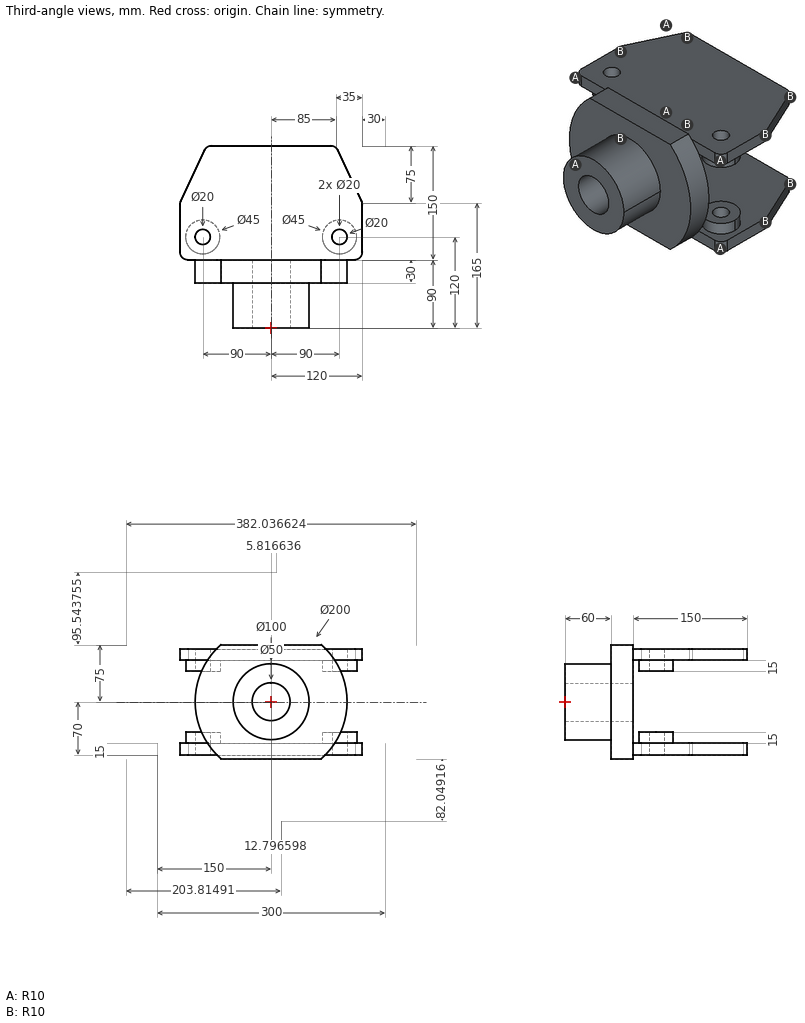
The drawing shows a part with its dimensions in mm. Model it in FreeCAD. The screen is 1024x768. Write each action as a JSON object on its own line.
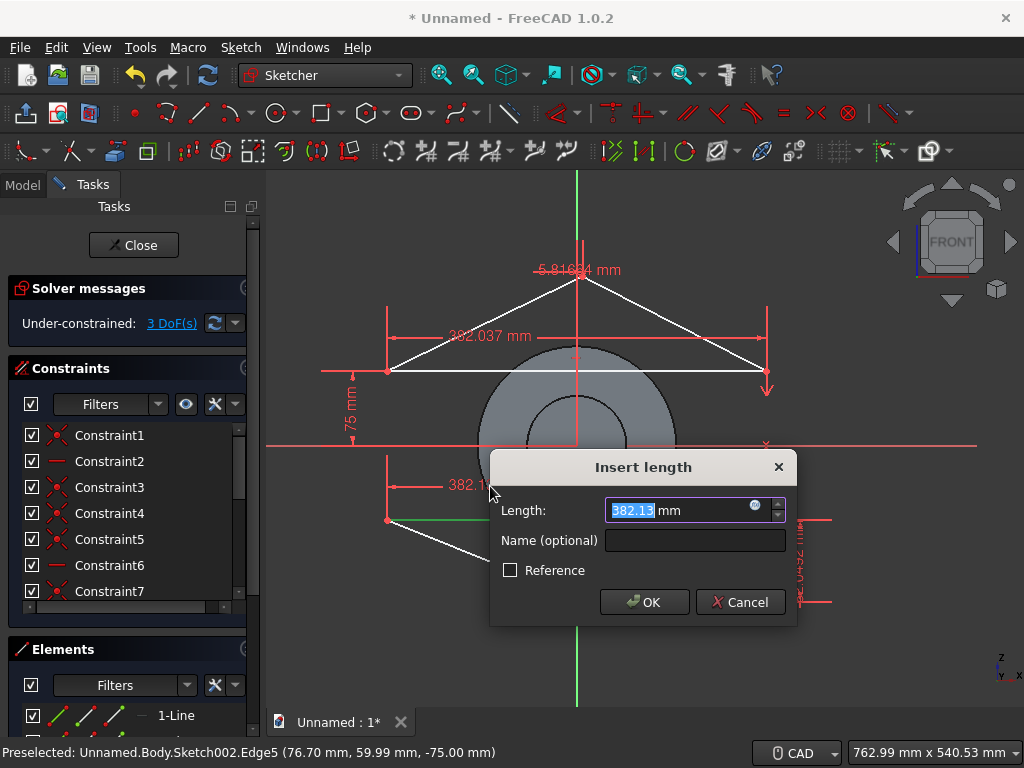
{"action": "type", "text": "382.036624"}
{"action": "key", "text": "Return"}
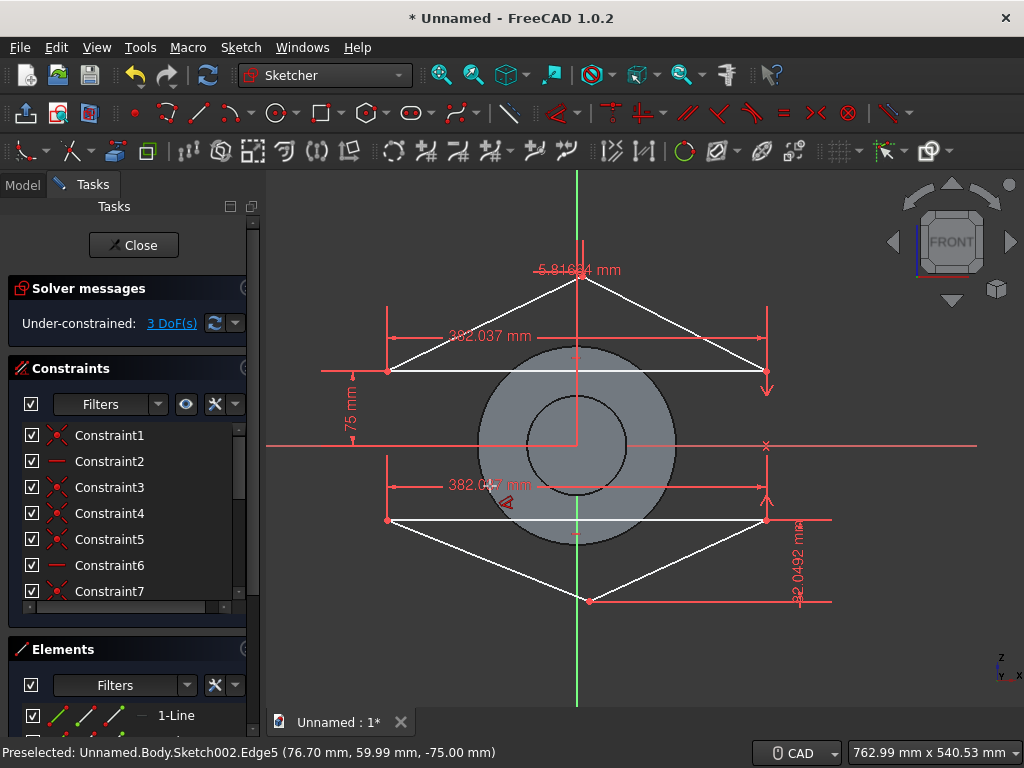
{"action": "scroll", "coordinate": [589, 602], "scroll_direction": "up", "scroll_amount": 6}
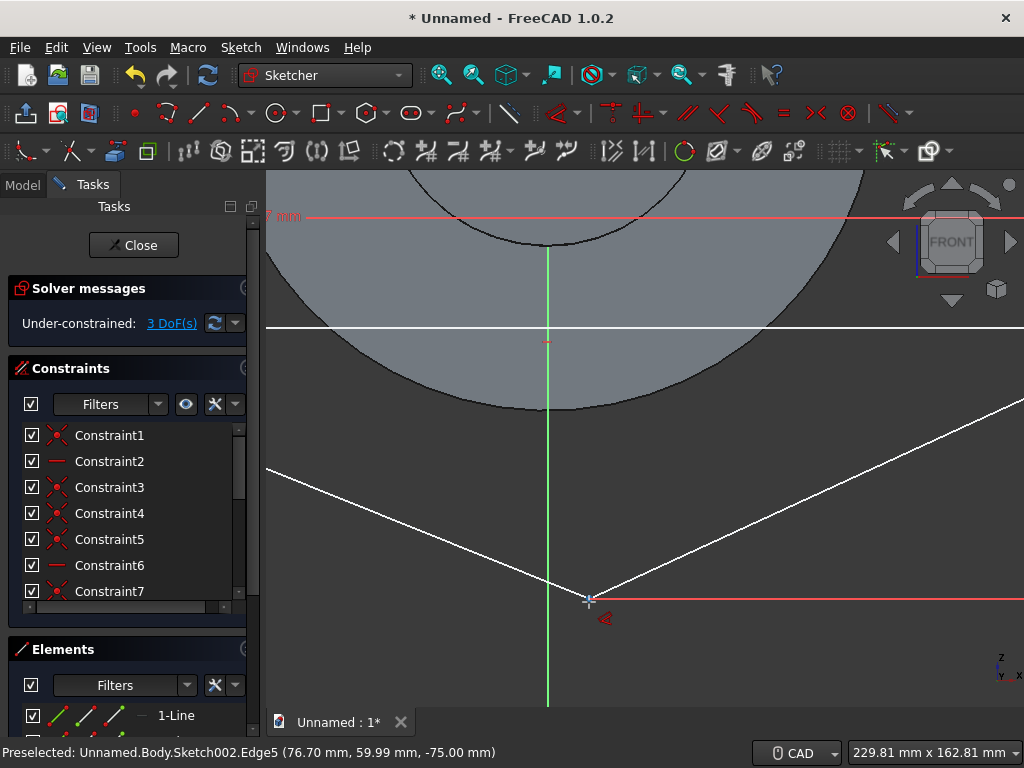
{"action": "left_click", "coordinate": [590, 599]}
{"action": "left_click", "coordinate": [569, 633]}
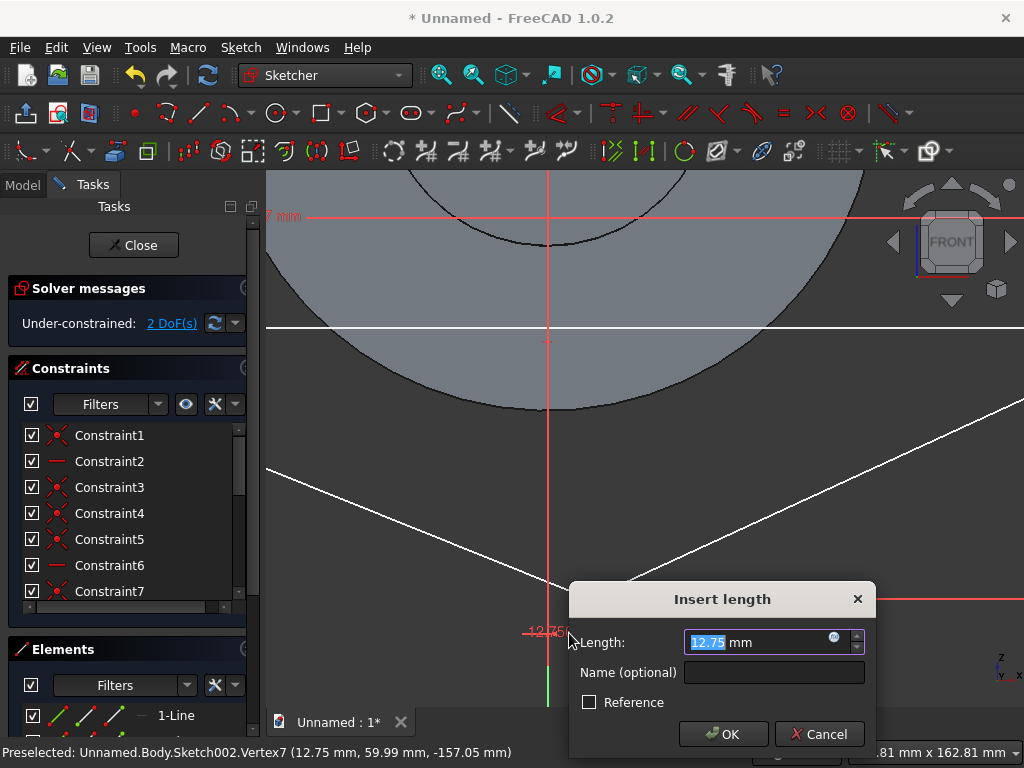
{"action": "type", "text": "12.796598"}
{"action": "key", "text": "Return"}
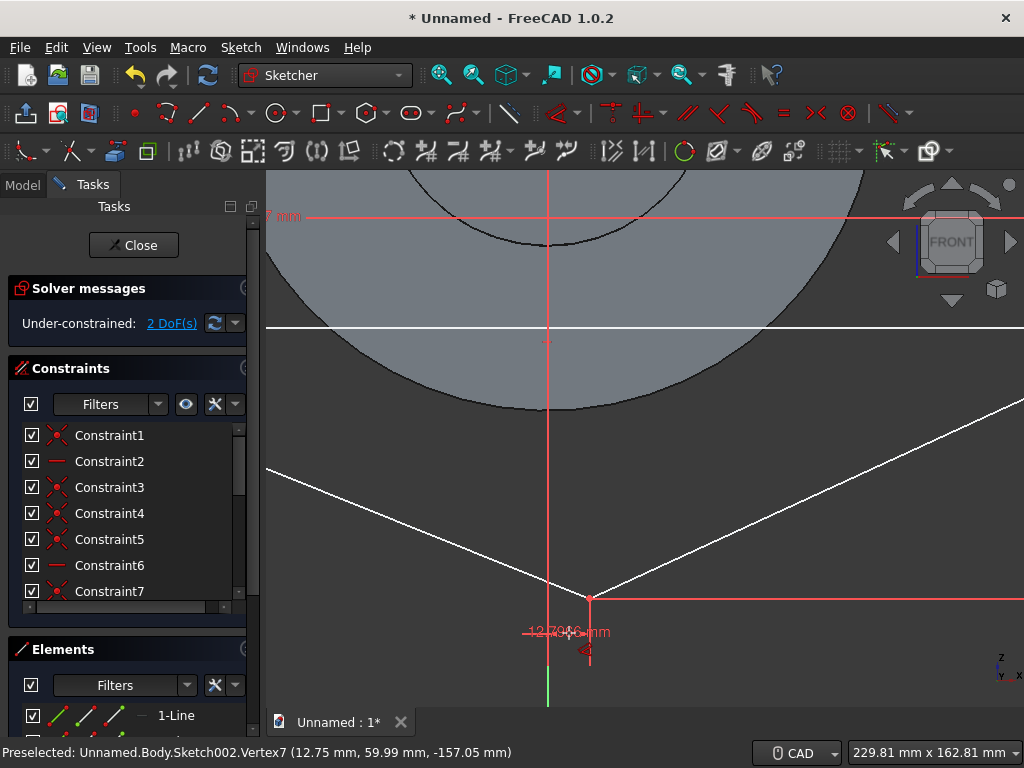
{"action": "scroll", "coordinate": [589, 602], "scroll_direction": "down", "scroll_amount": 6}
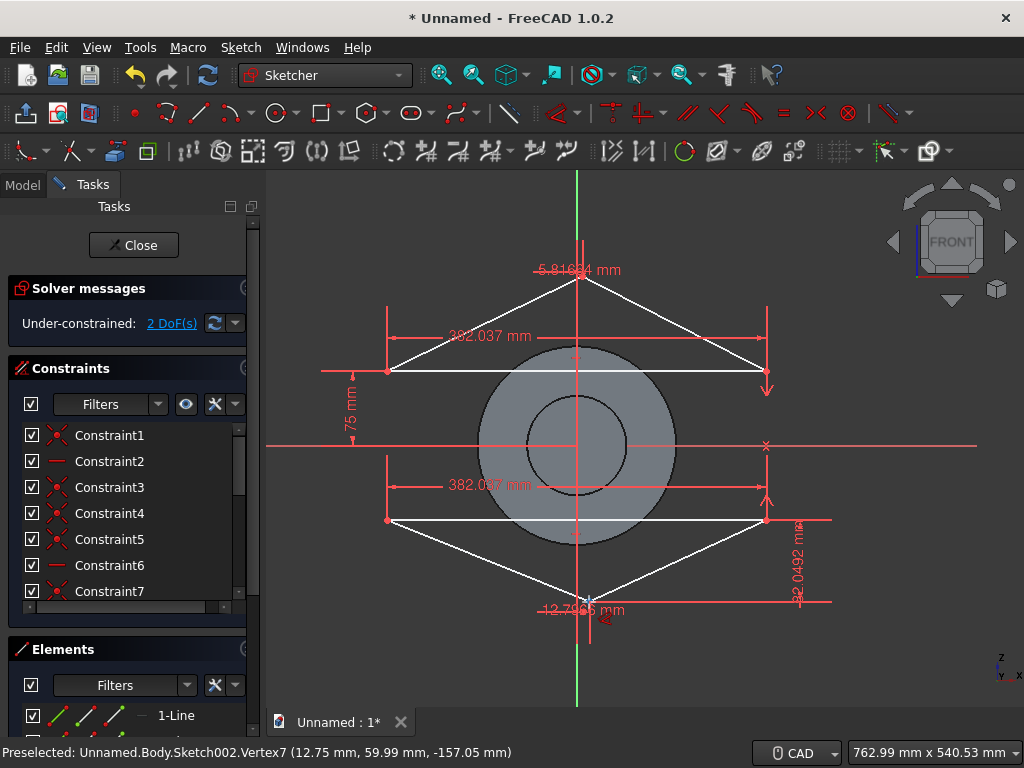
{"action": "left_click", "coordinate": [524, 305]}
{"action": "left_click", "coordinate": [353, 324]}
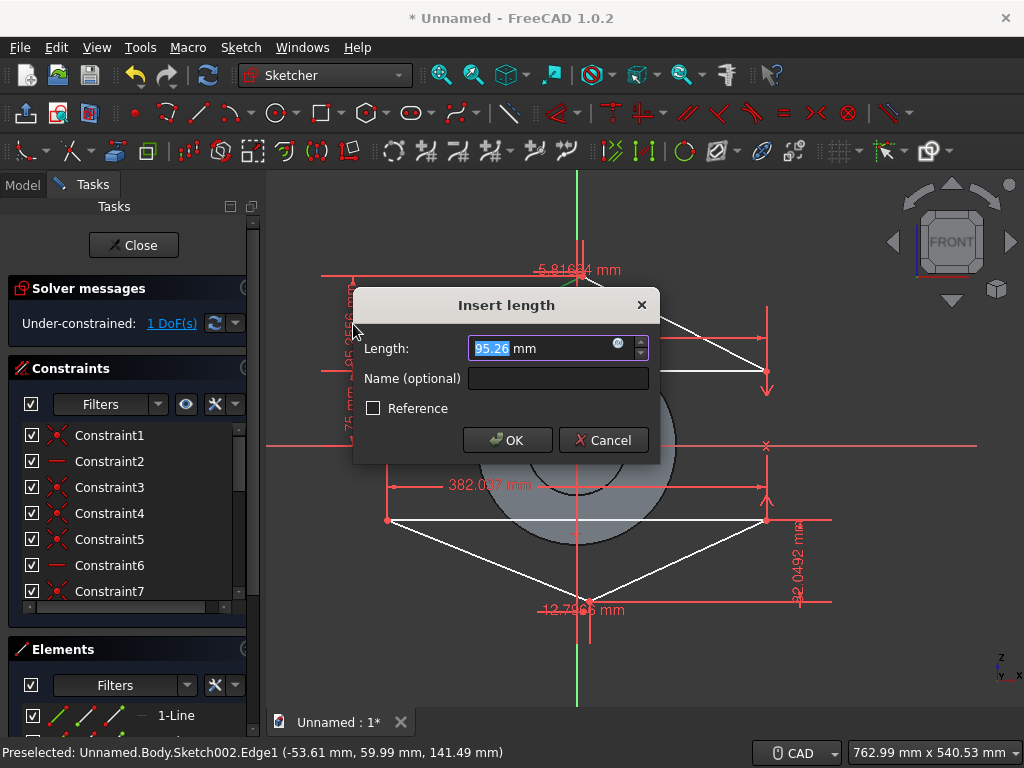
{"action": "type", "text": "95.543755"}
{"action": "key", "text": "Return"}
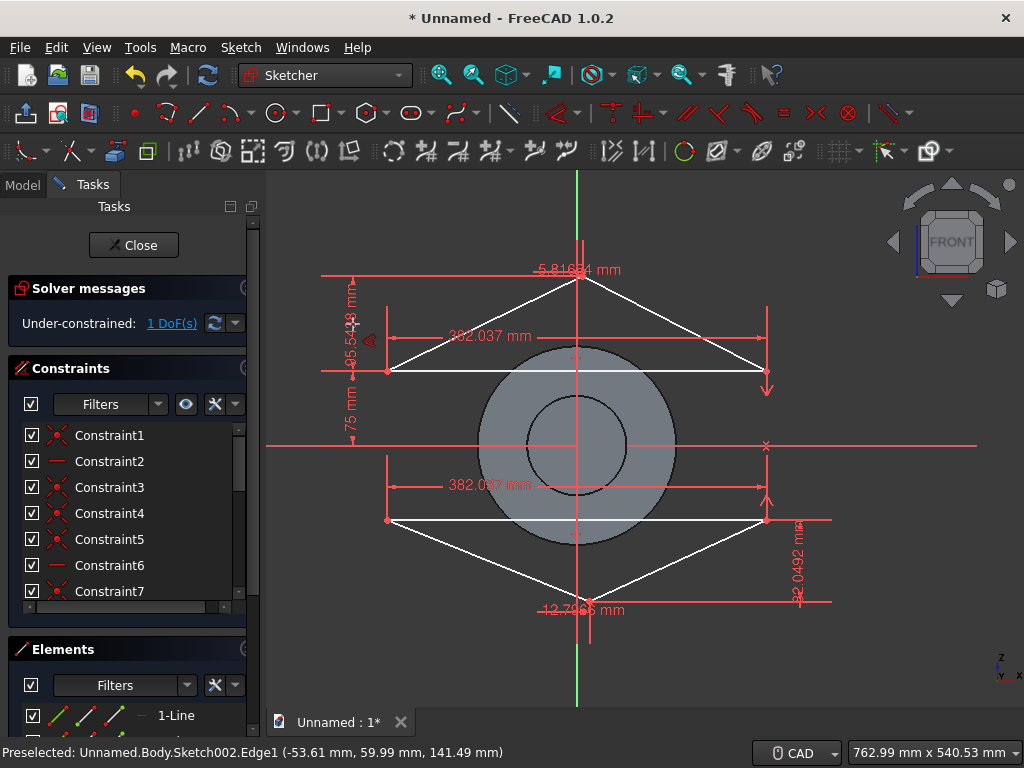
{"action": "left_click", "coordinate": [448, 545]}
{"action": "left_click", "coordinate": [488, 636]}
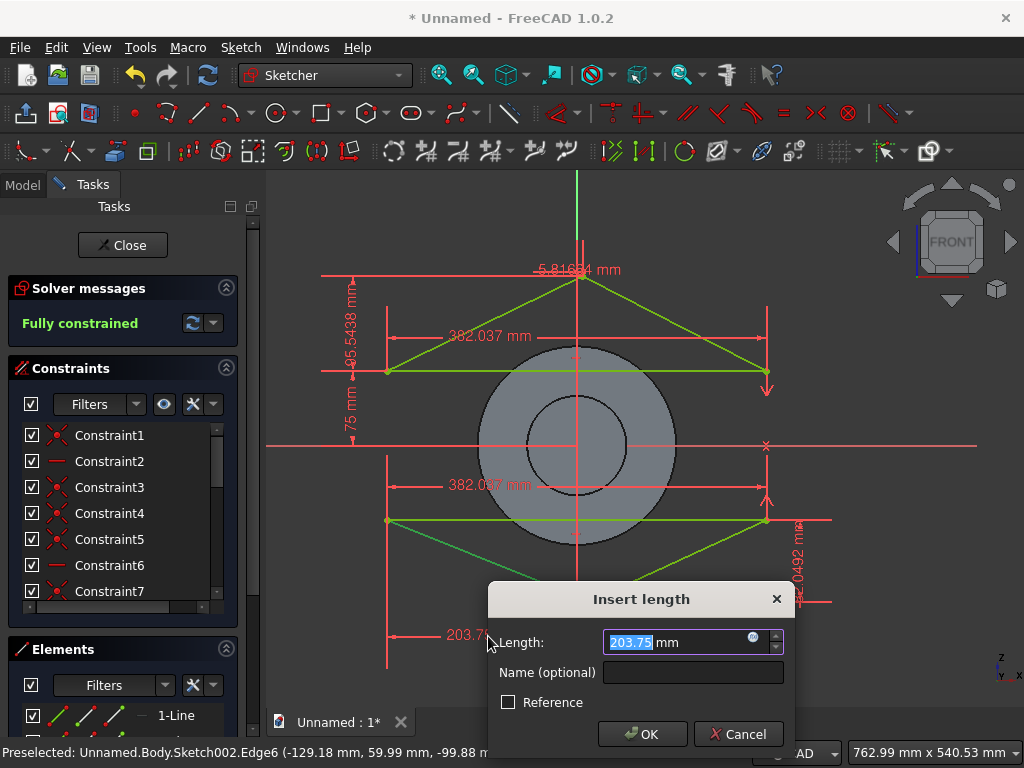
{"action": "type", "text": "203.81491"}
{"action": "key", "text": "Return"}
{"action": "key", "text": "Escape"}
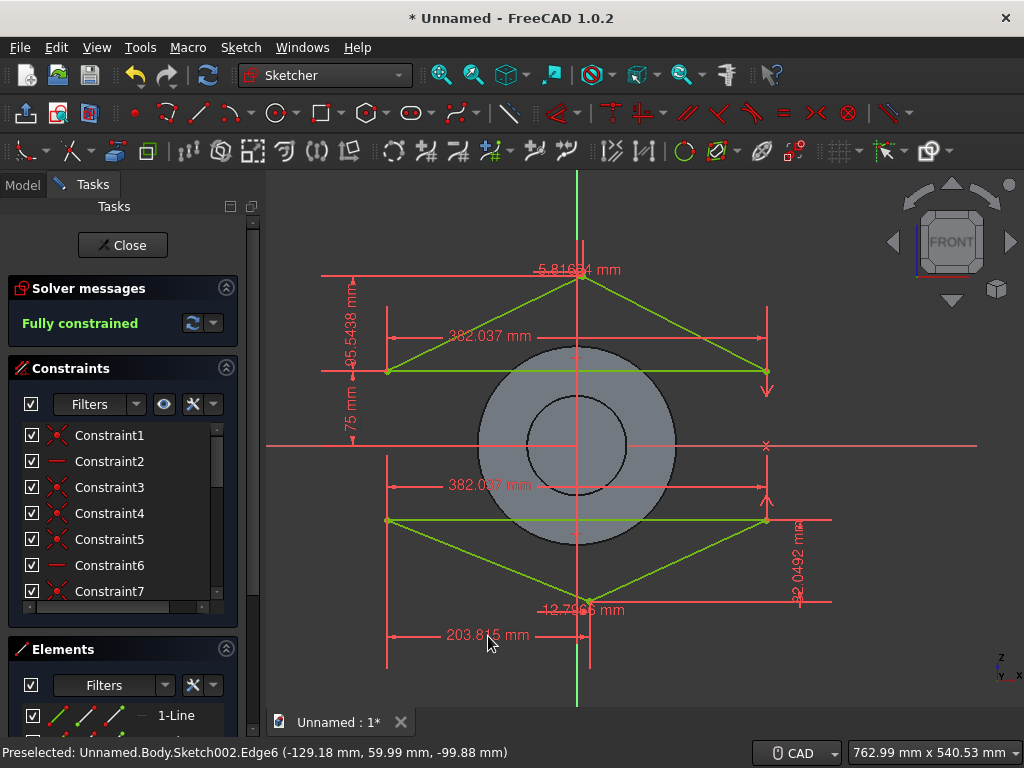
{"action": "left_click", "coordinate": [123, 245]}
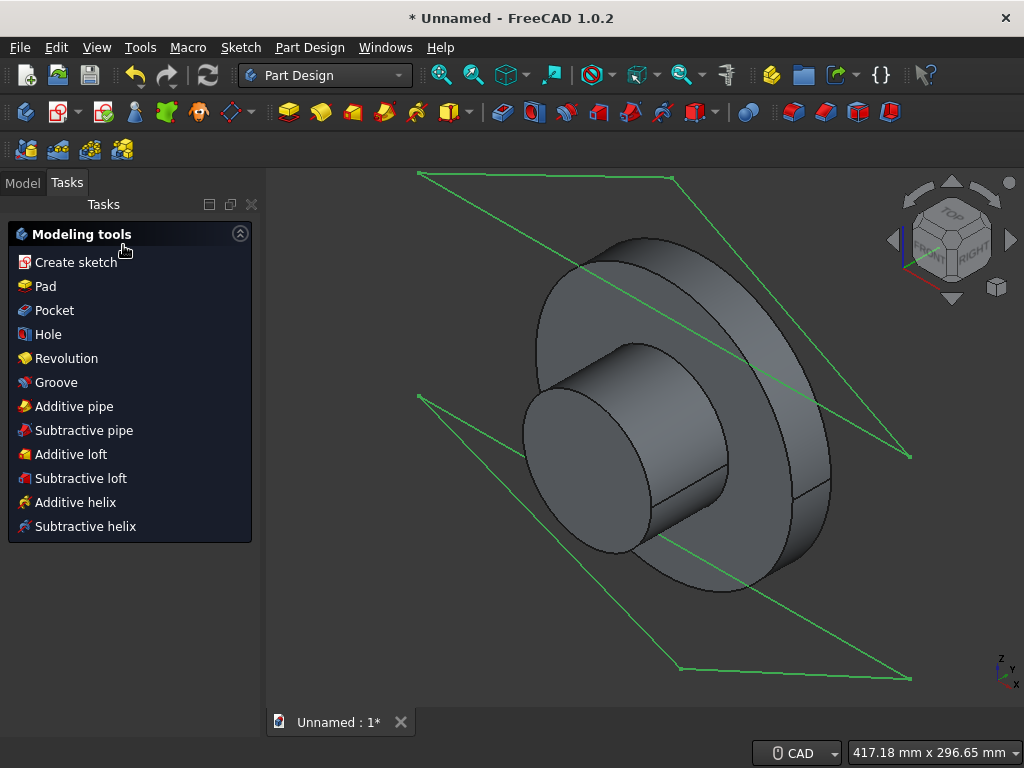
{"action": "left_click", "coordinate": [504, 112]}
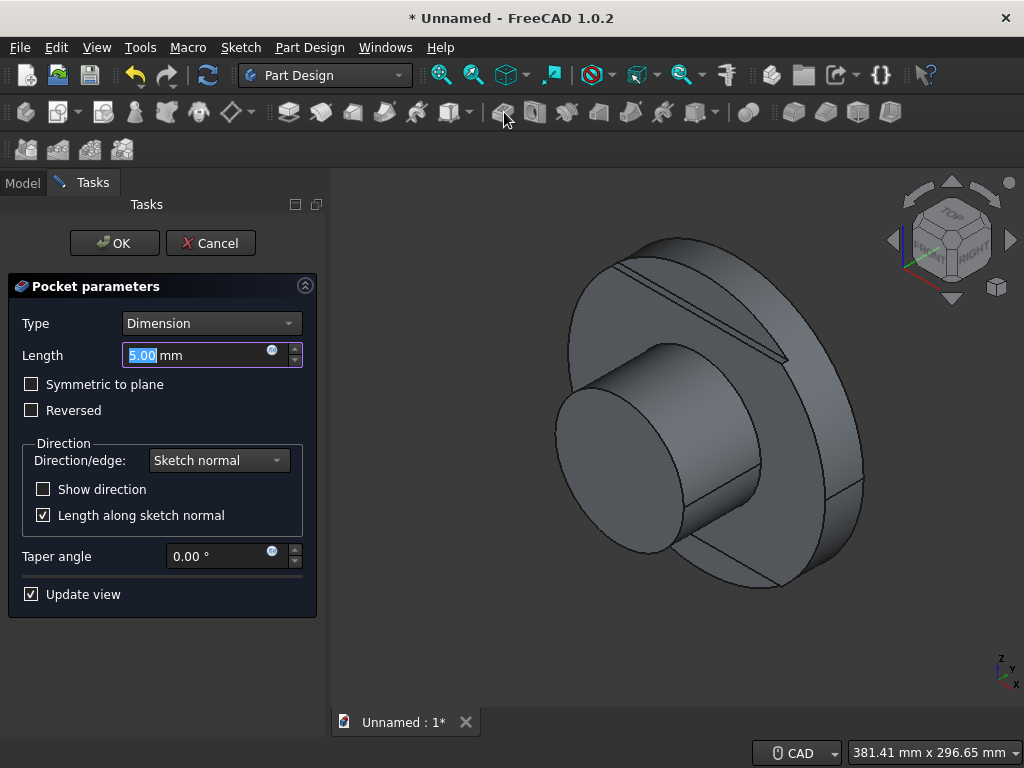
{"action": "left_click", "coordinate": [212, 324]}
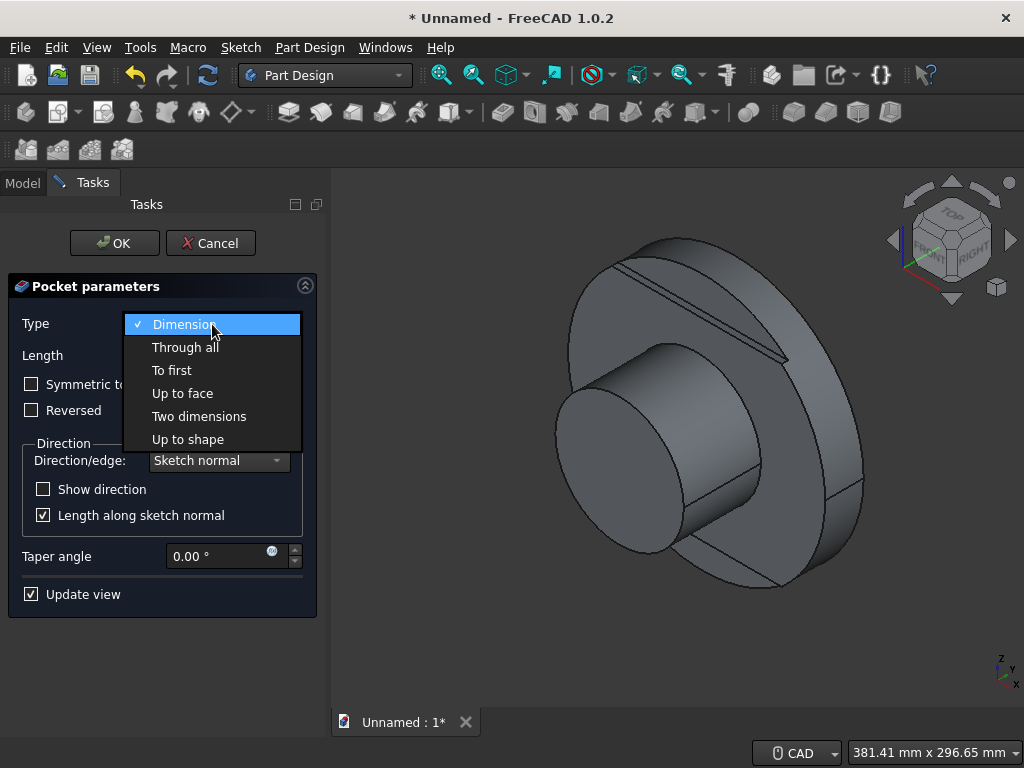
{"action": "left_click", "coordinate": [212, 348]}